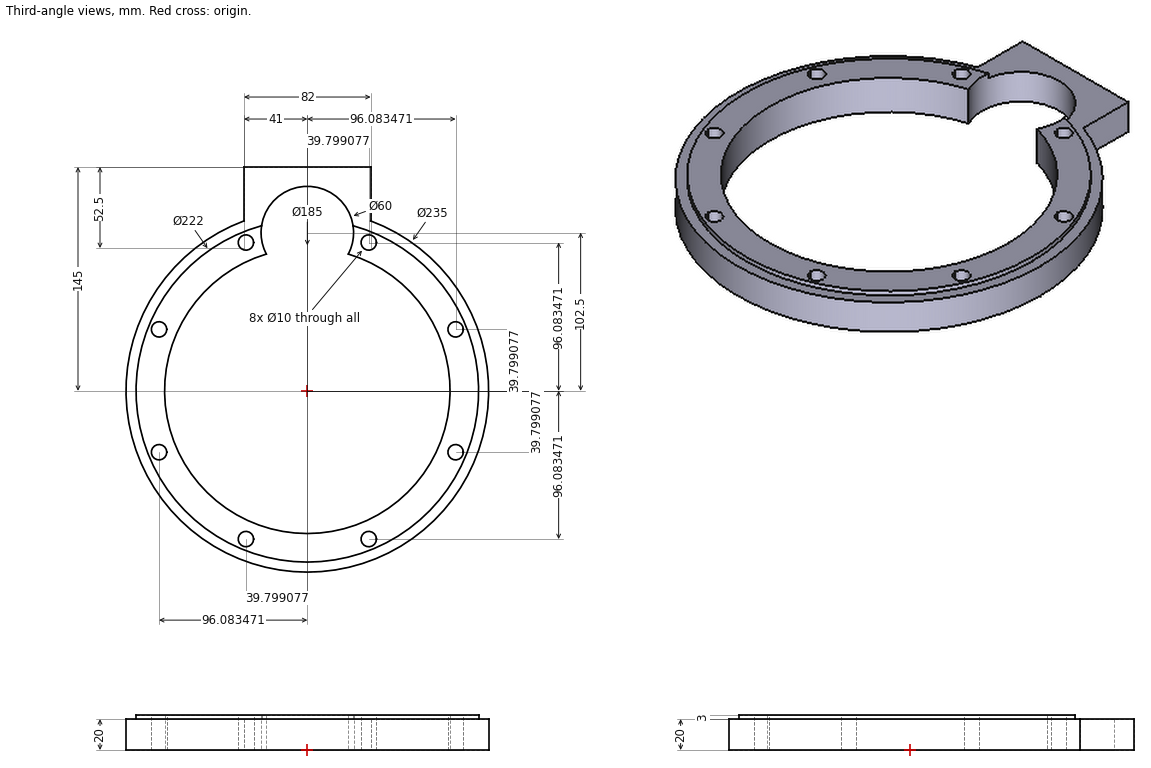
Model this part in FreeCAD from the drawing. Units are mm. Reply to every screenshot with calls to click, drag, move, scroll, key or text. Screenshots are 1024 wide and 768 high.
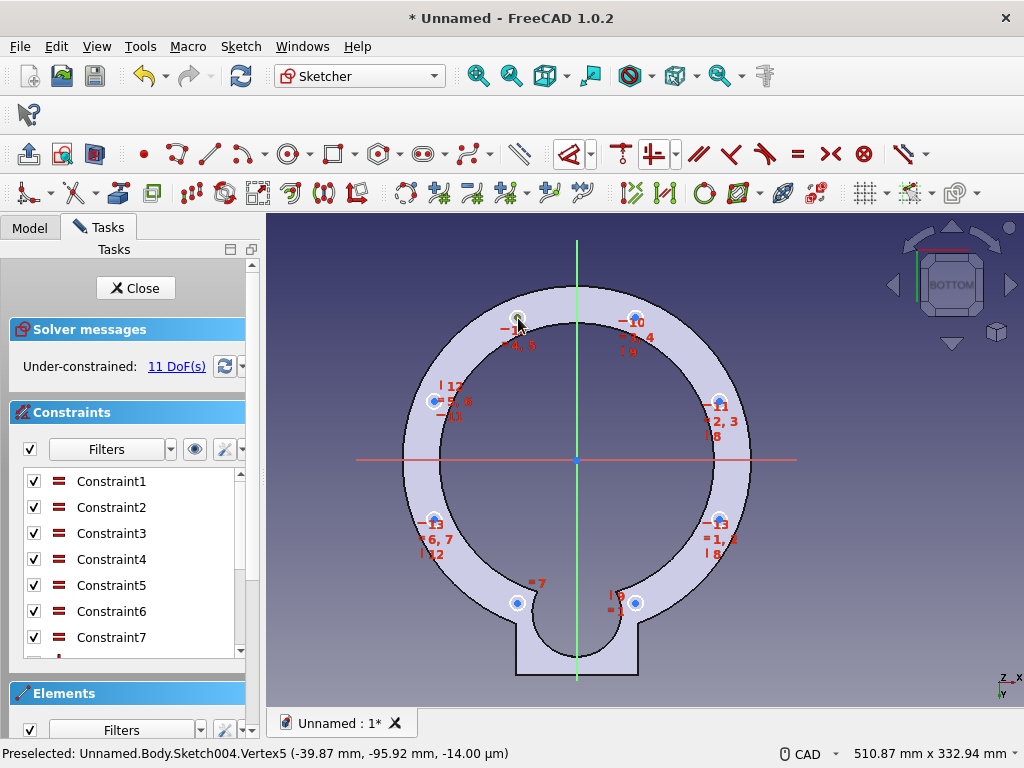
click(518, 603)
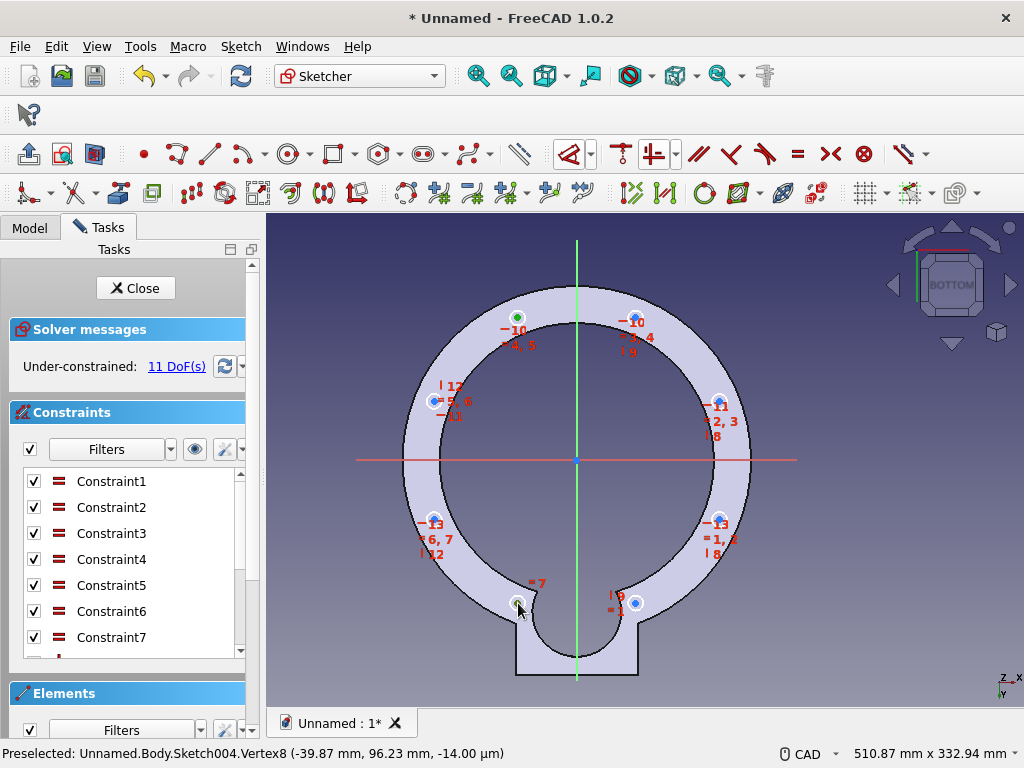
click(676, 154)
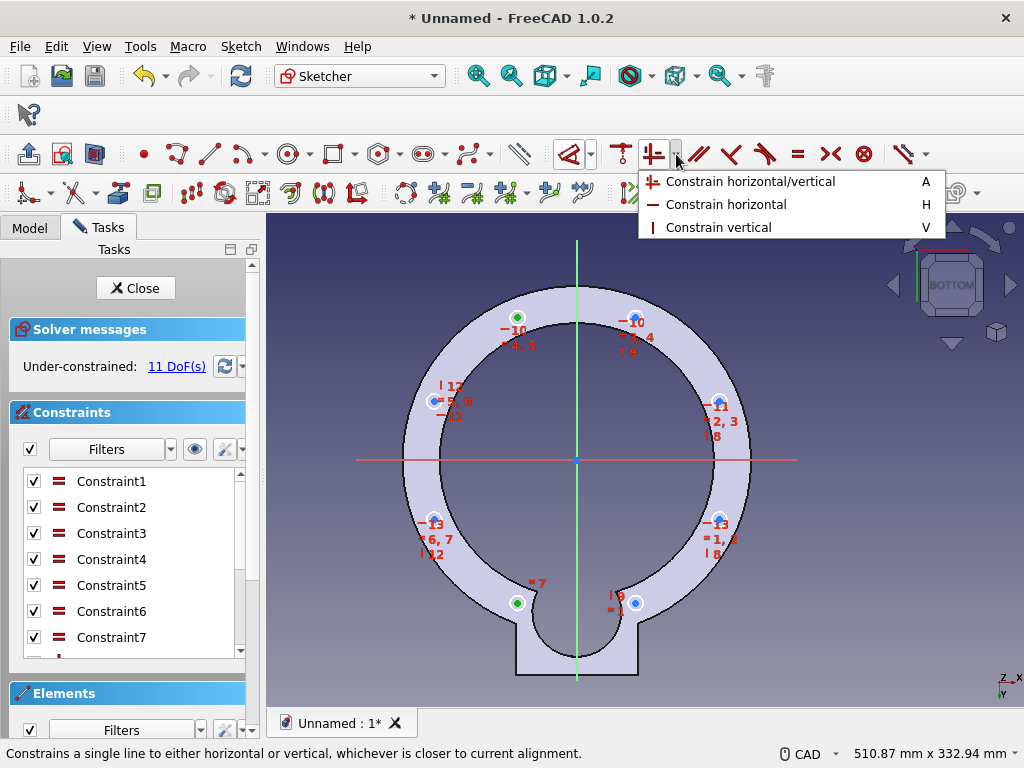
click(792, 228)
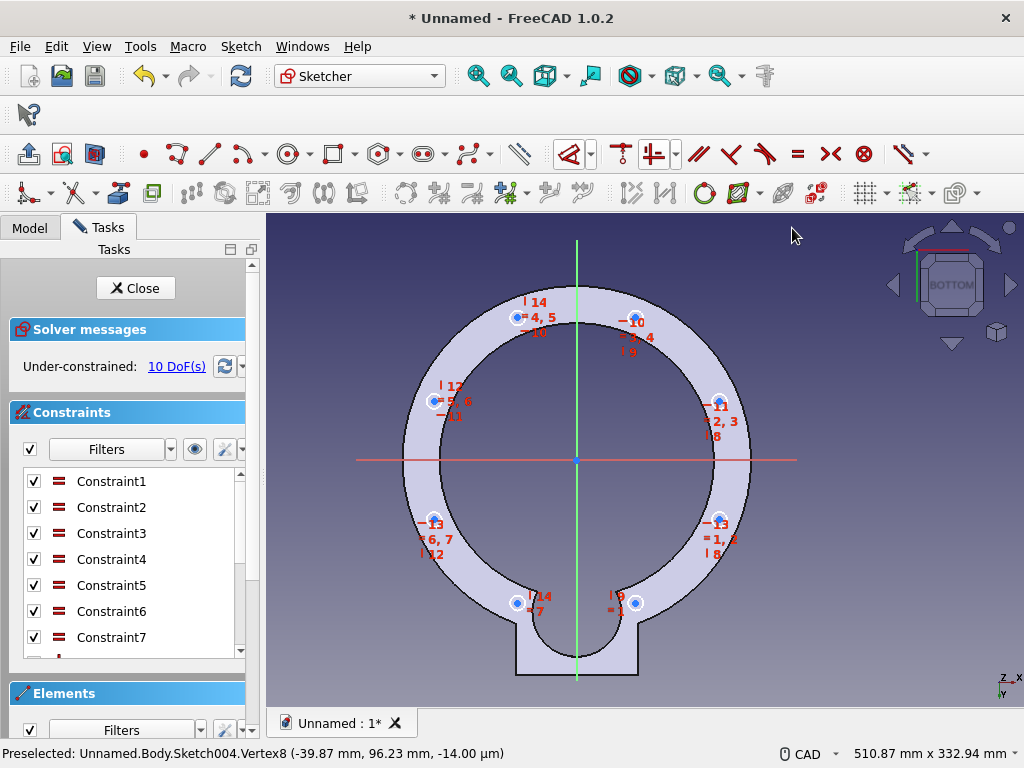
click(636, 603)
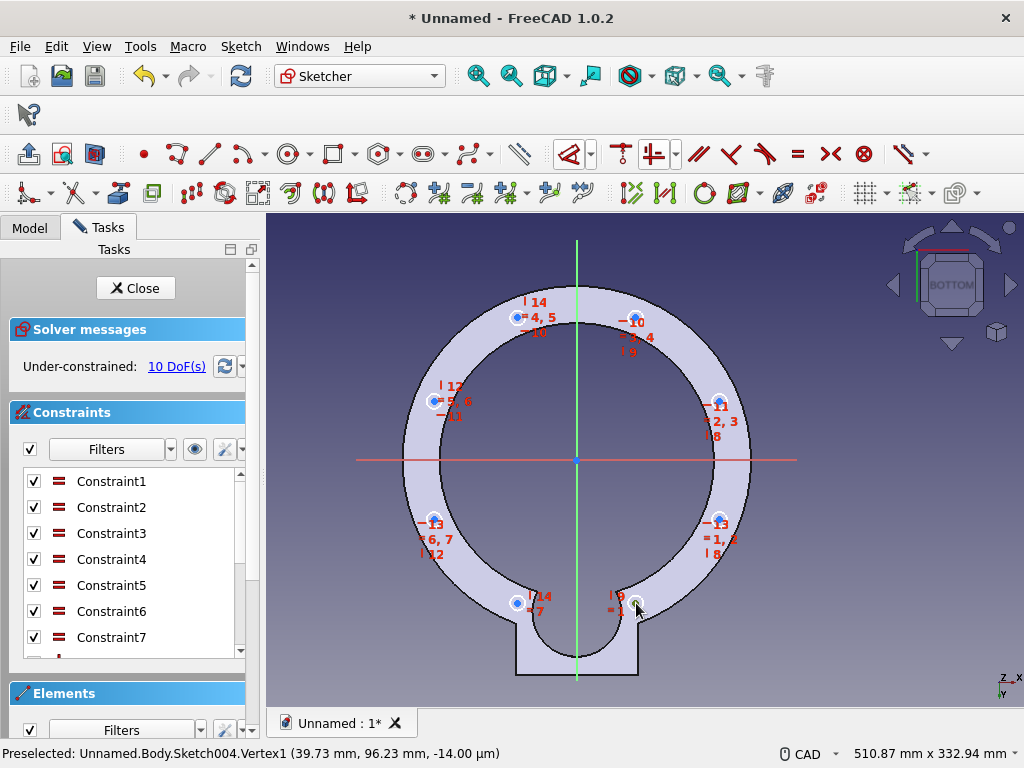
click(518, 603)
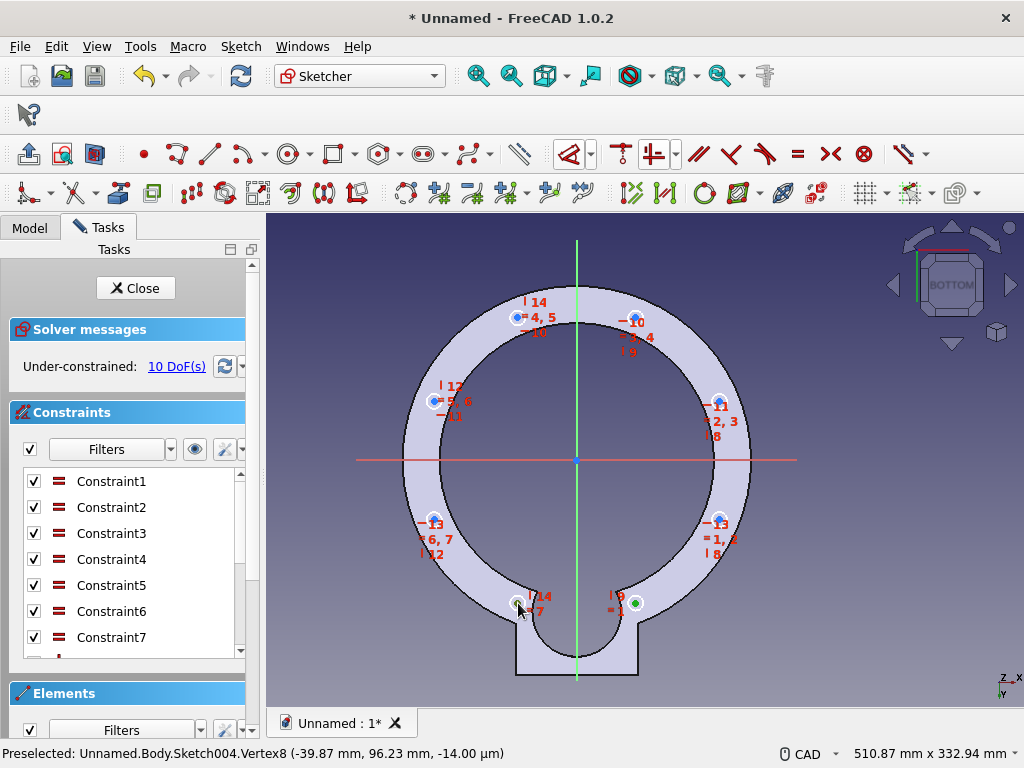
click(676, 154)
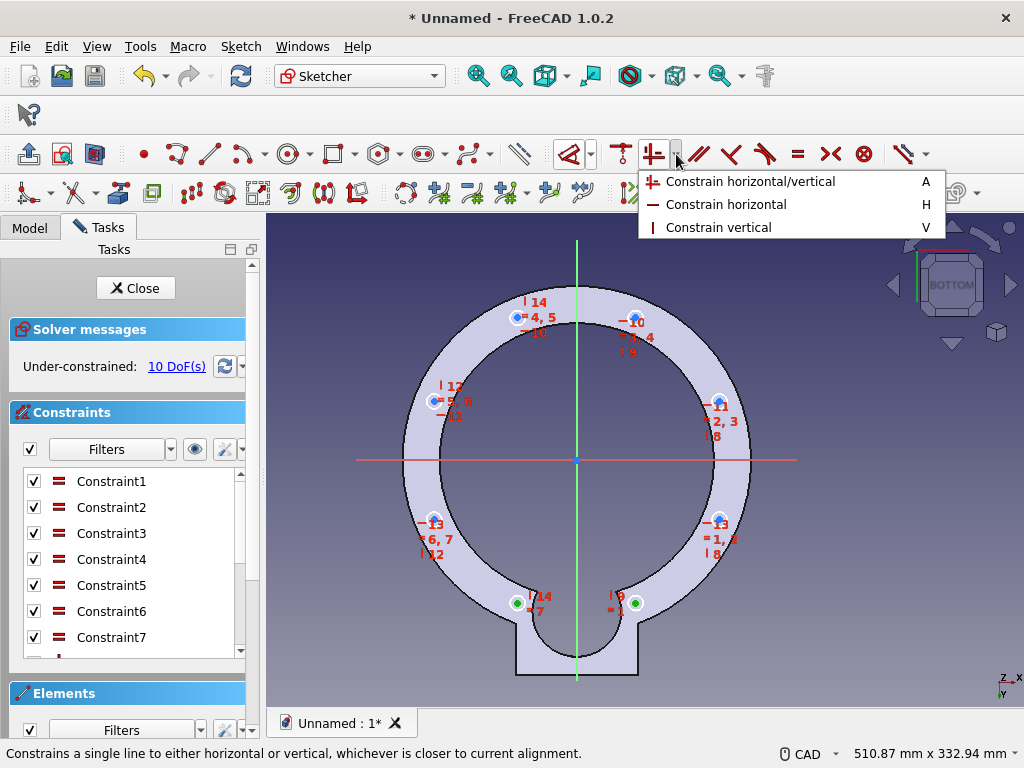
click(792, 204)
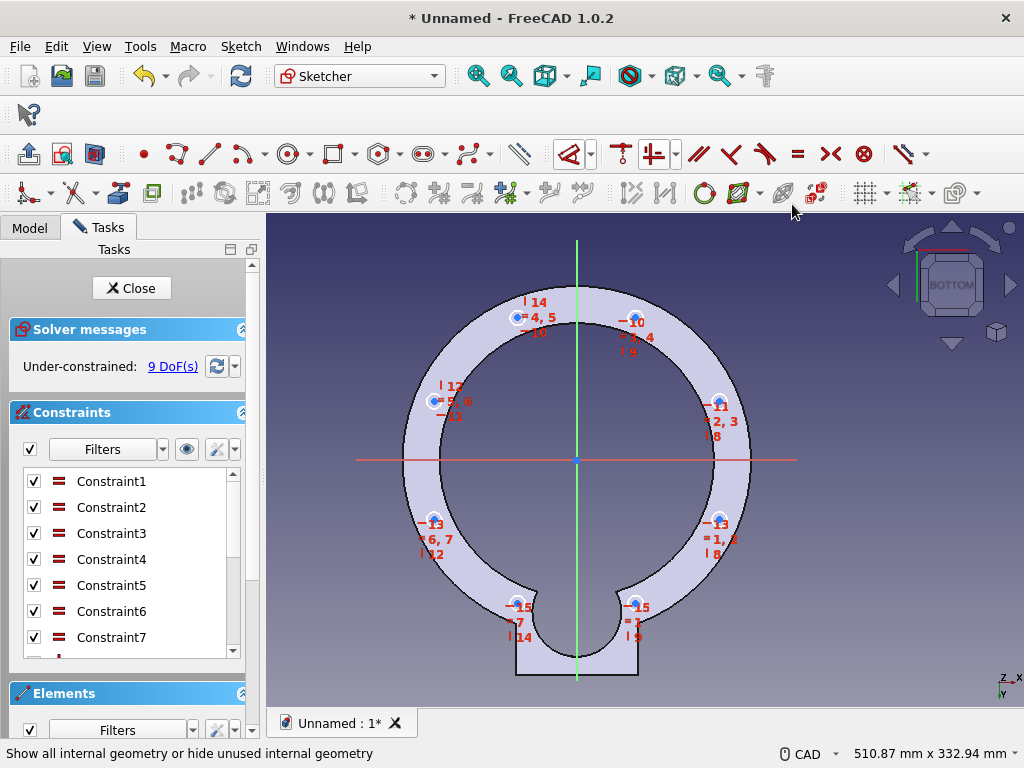
scroll(641, 598, up, 5)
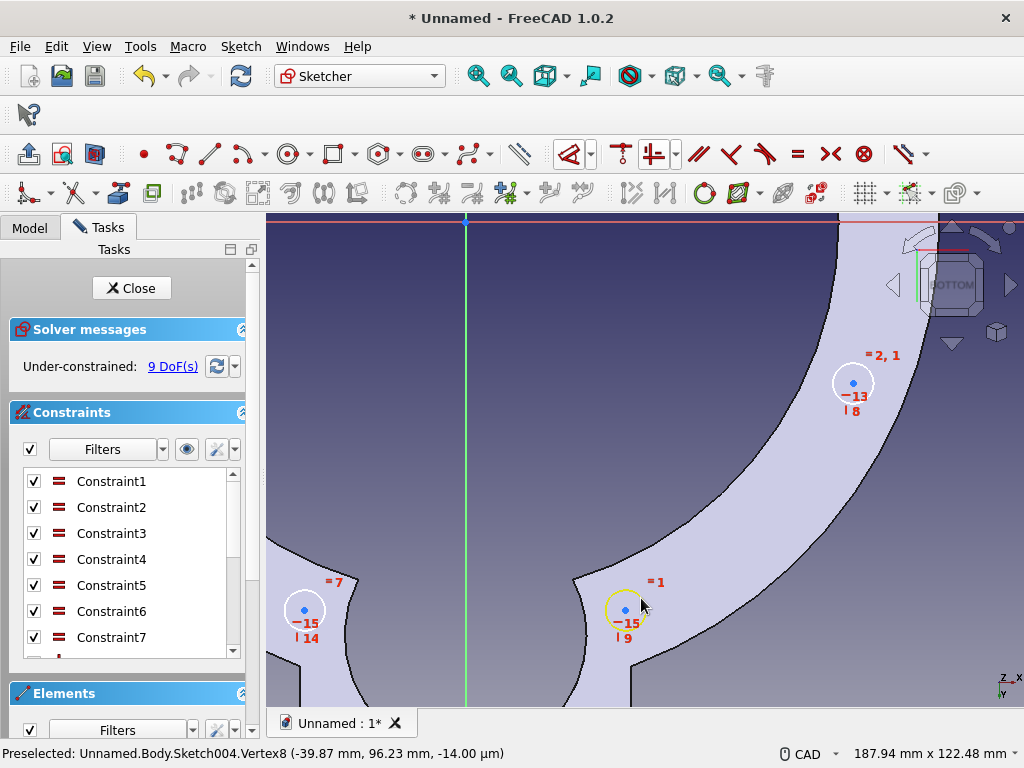
click(640, 596)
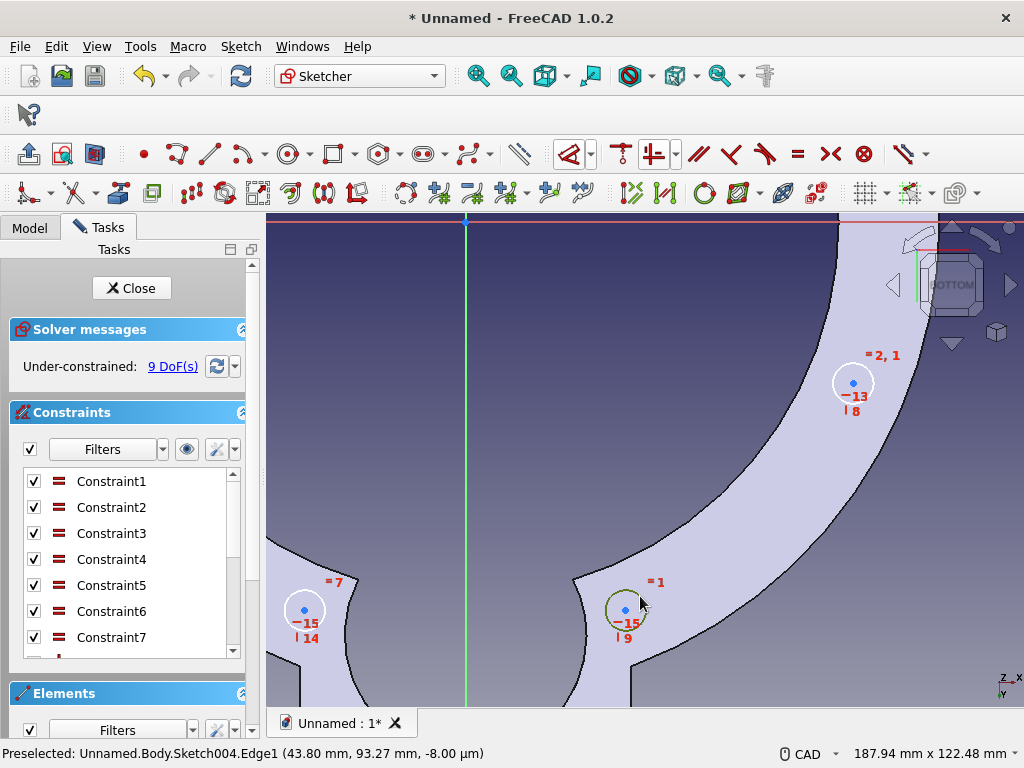
click(590, 154)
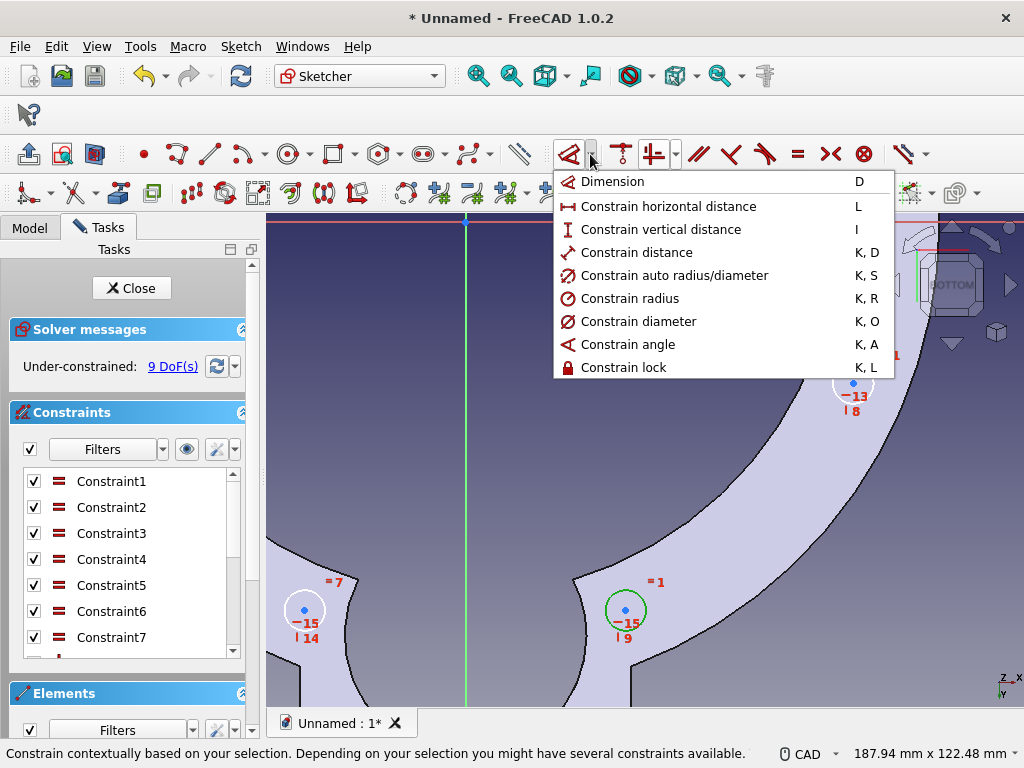
click(724, 322)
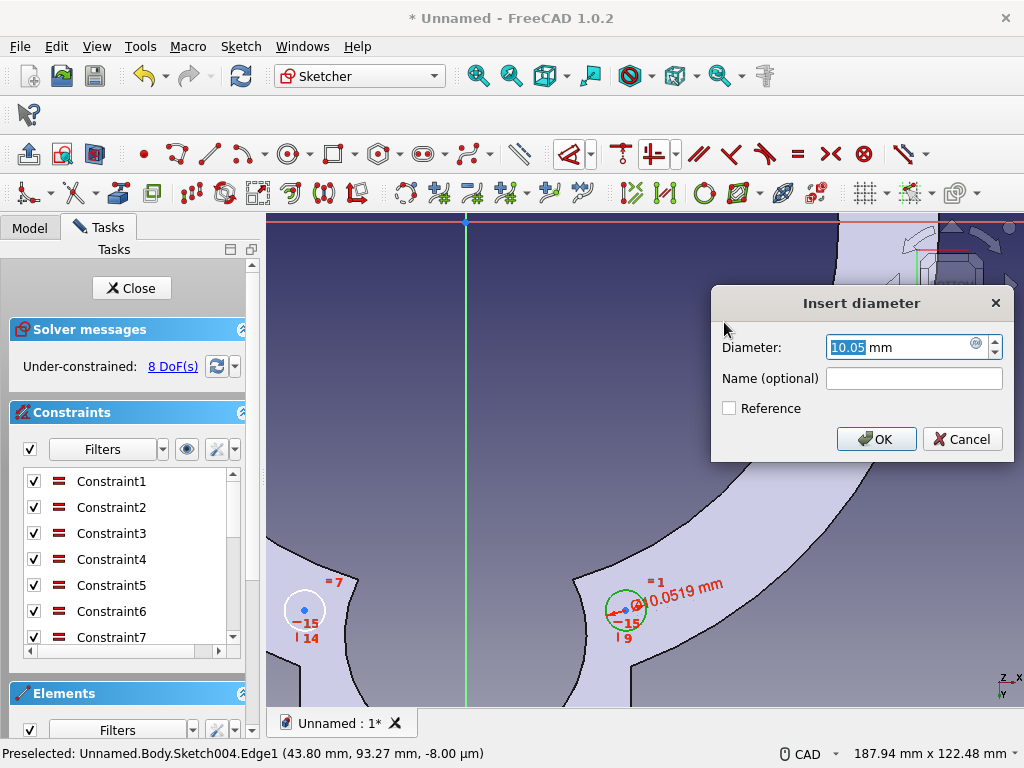
text(10)
key(Return)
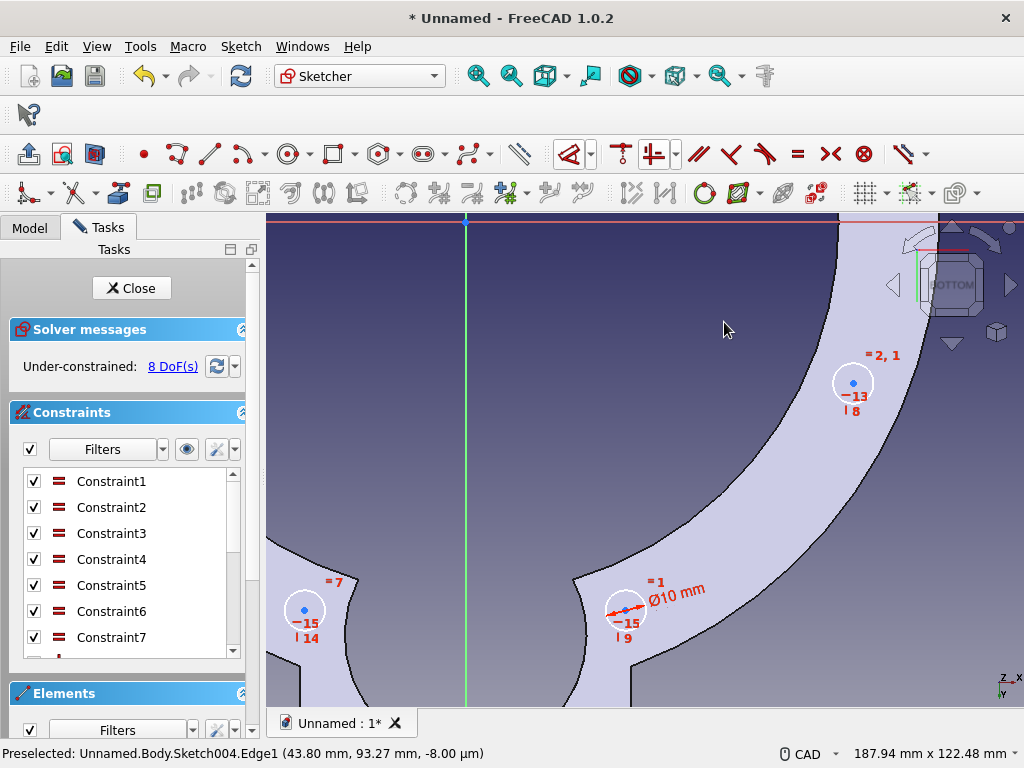
click(626, 610)